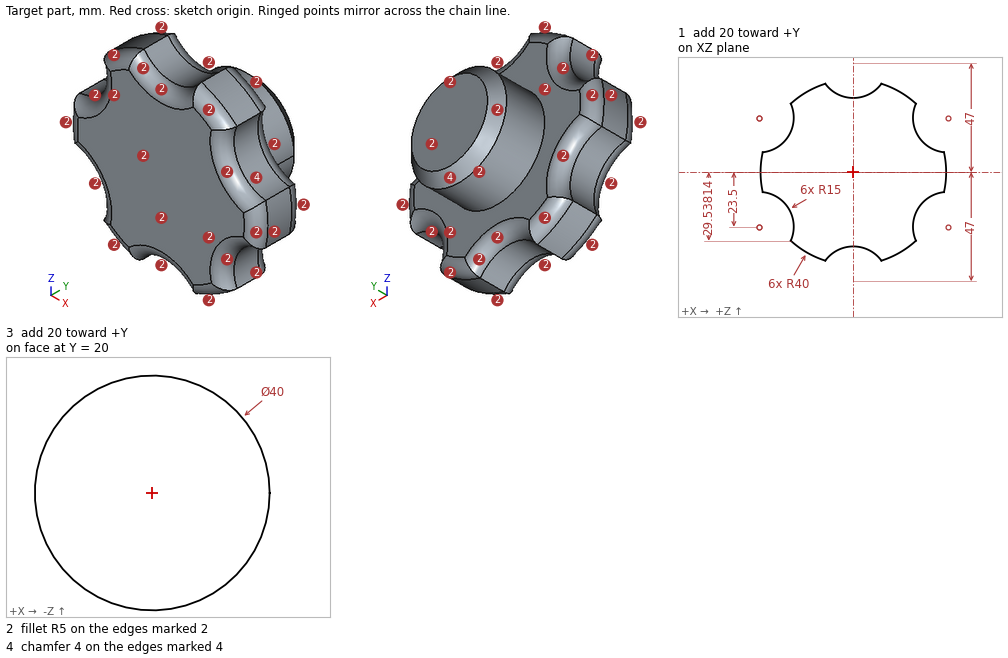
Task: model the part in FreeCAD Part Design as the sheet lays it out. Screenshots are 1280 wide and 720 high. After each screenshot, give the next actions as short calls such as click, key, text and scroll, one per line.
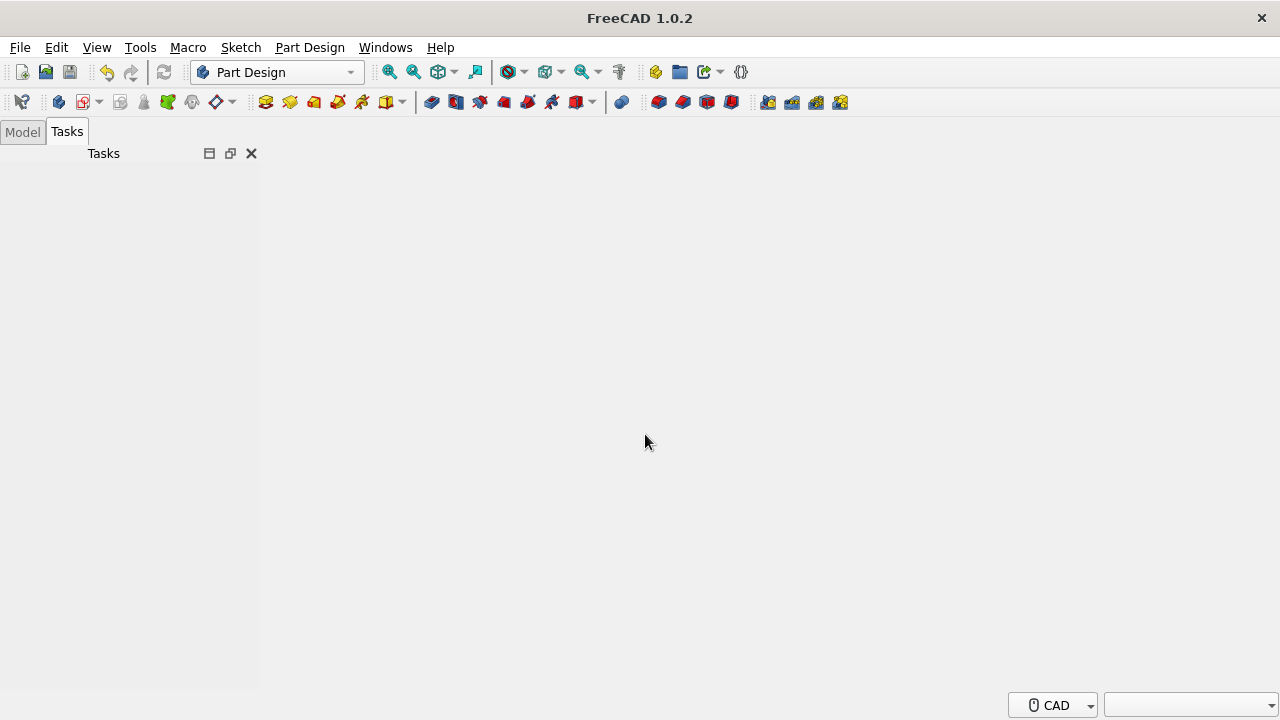
click(22, 72)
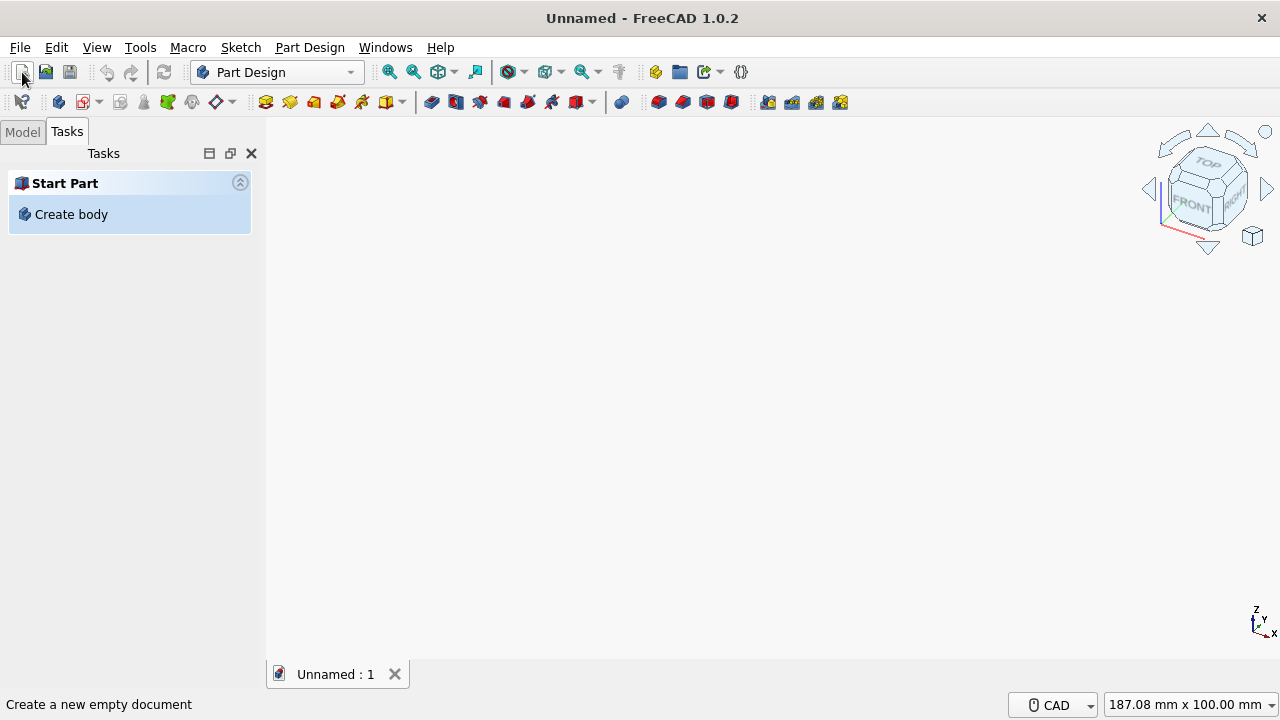
click(84, 102)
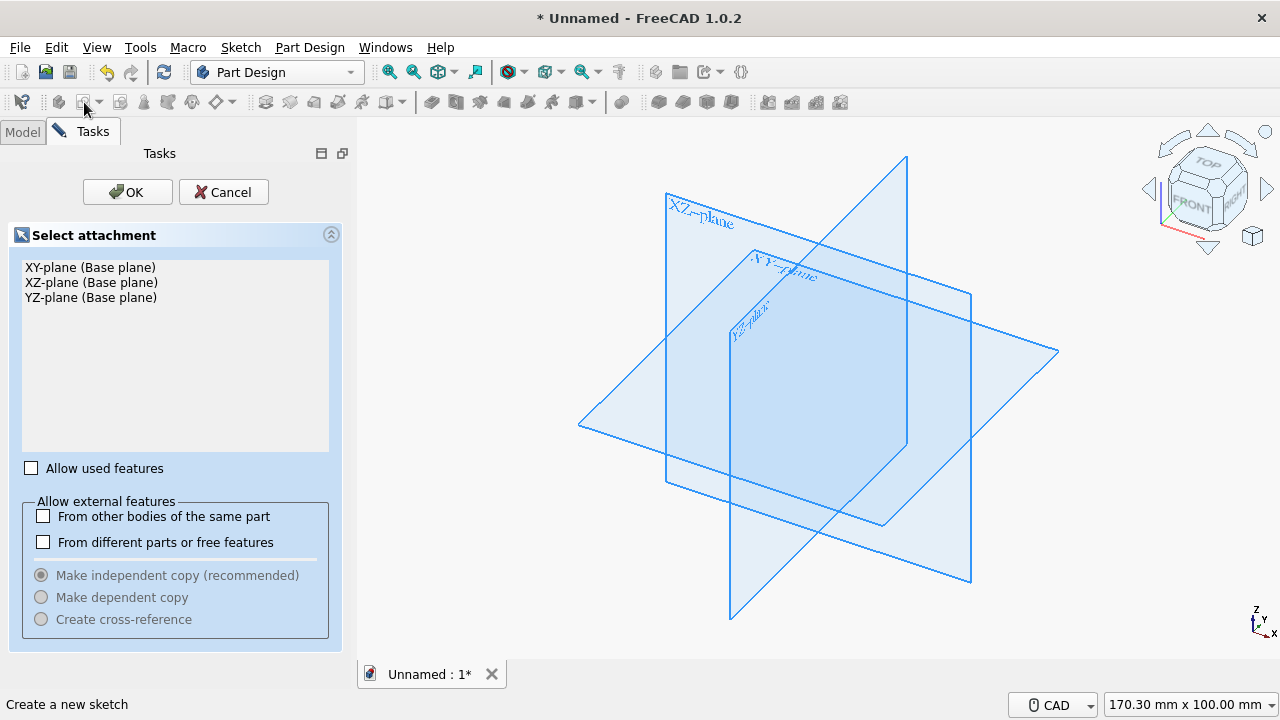
click(82, 282)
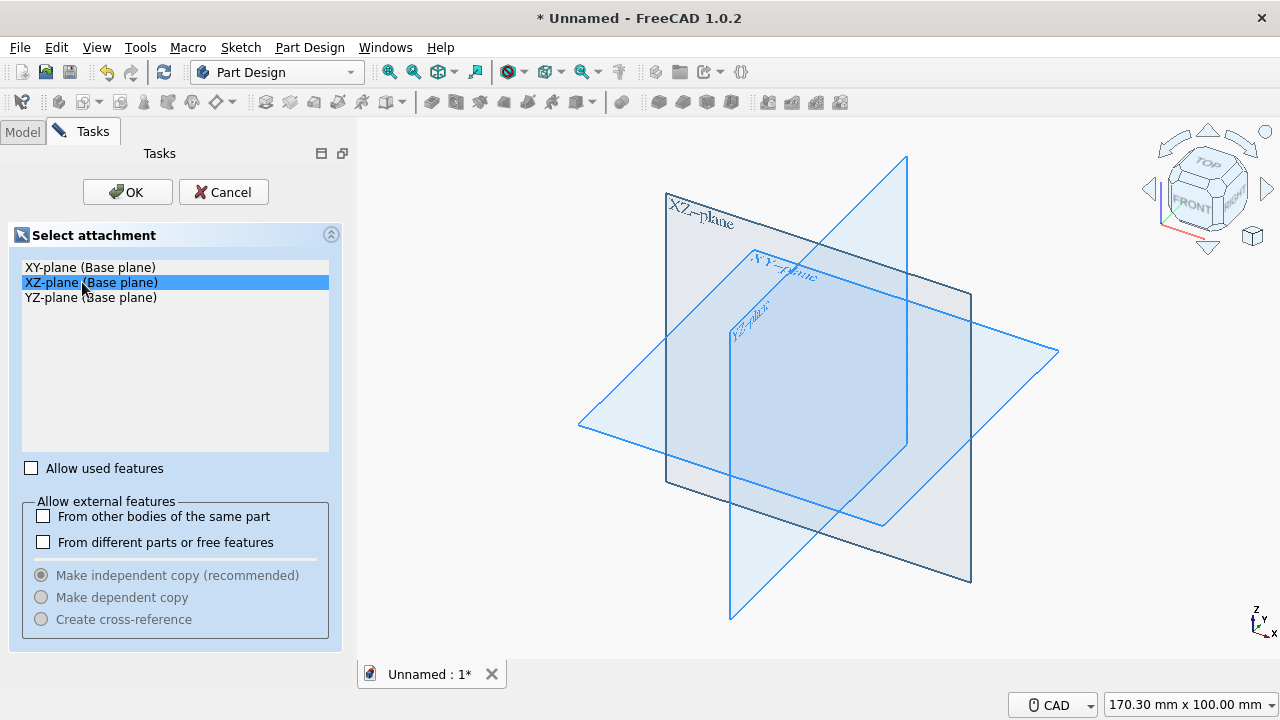
click(128, 192)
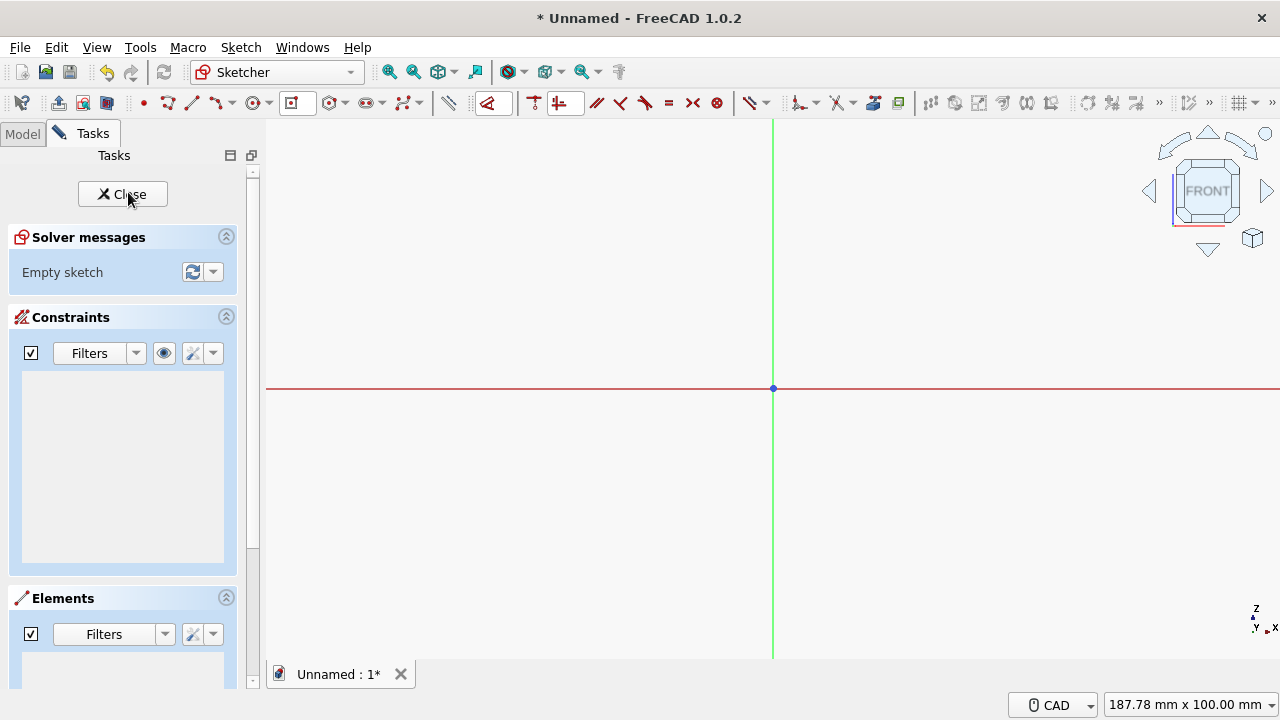
click(216, 104)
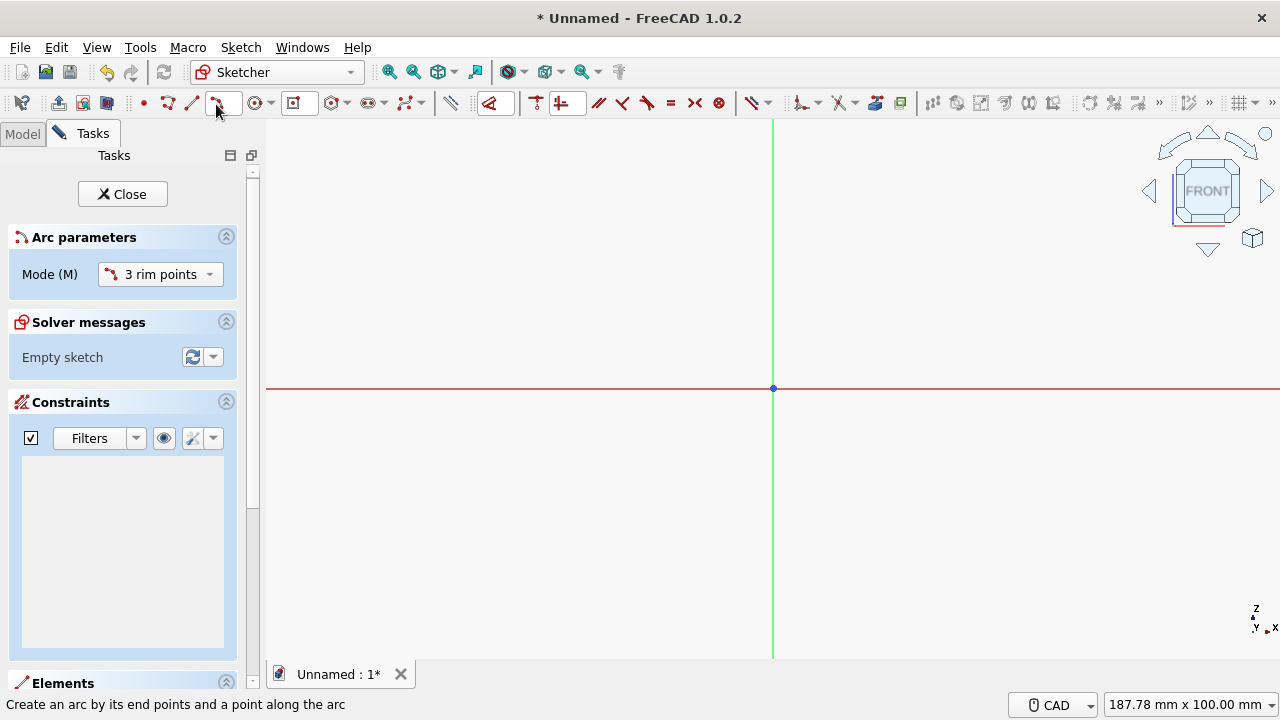
click(708, 595)
click(627, 549)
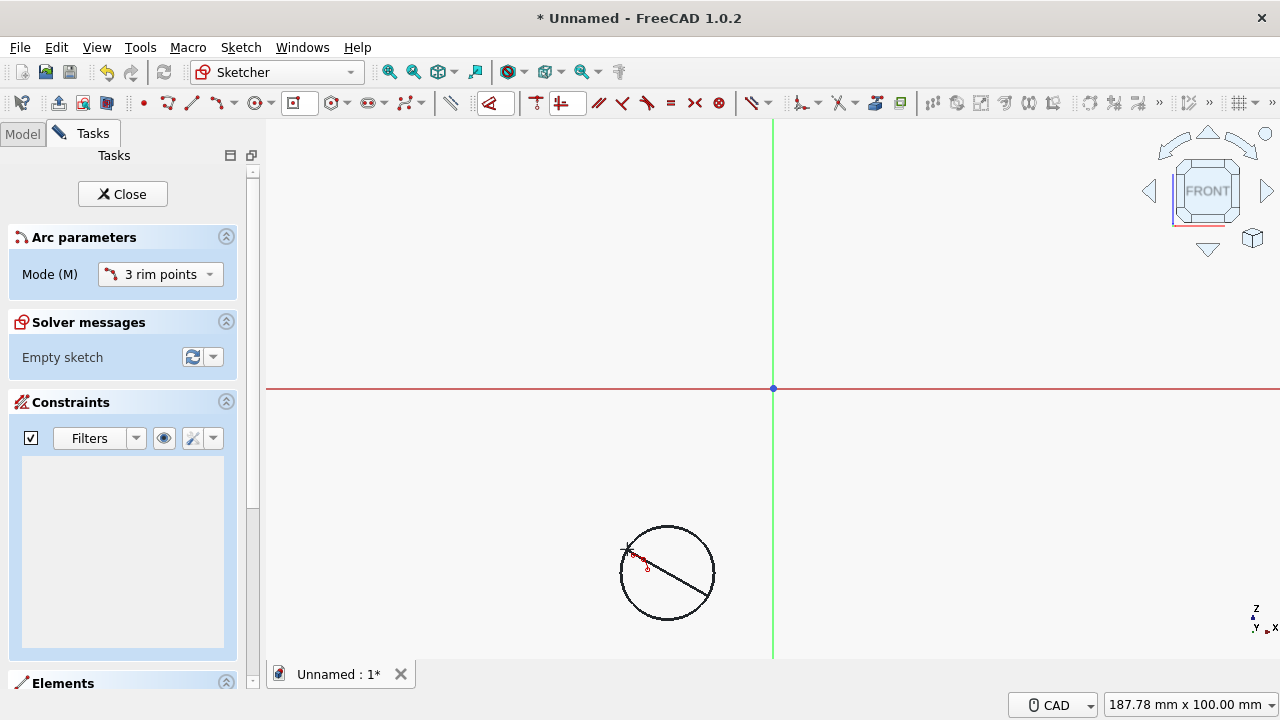
scroll(665, 576, up, 6)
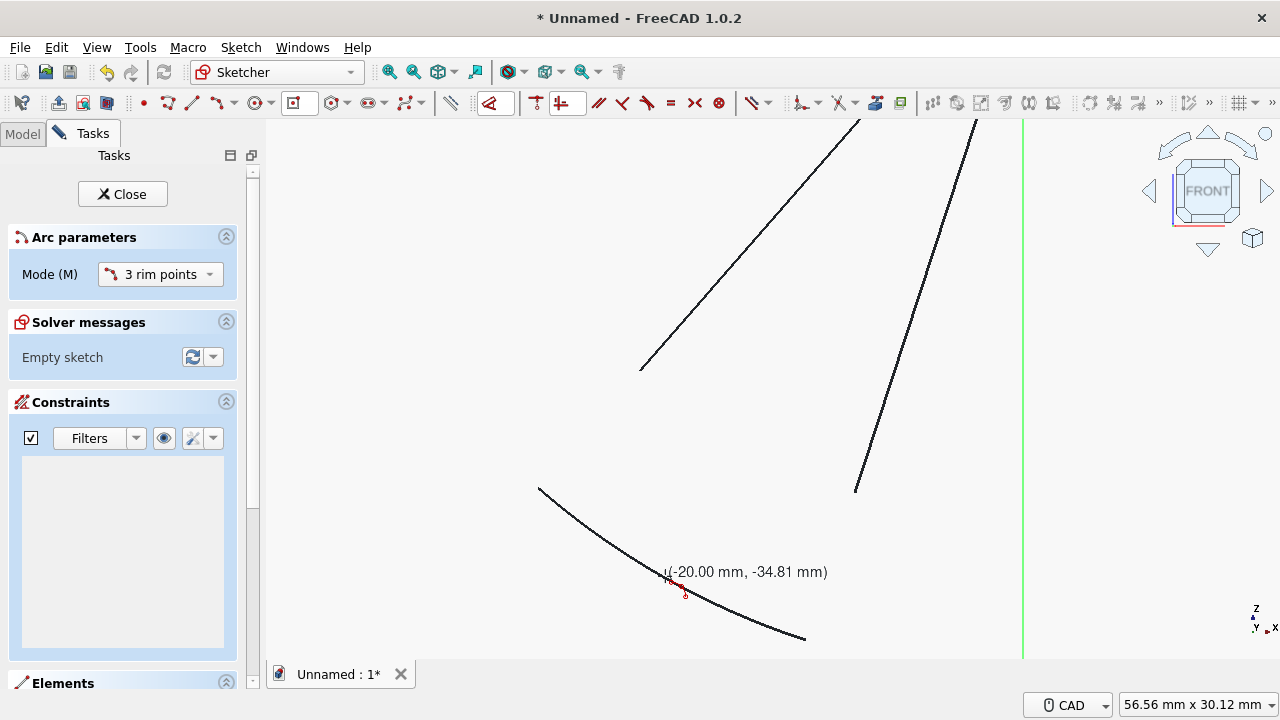
click(664, 574)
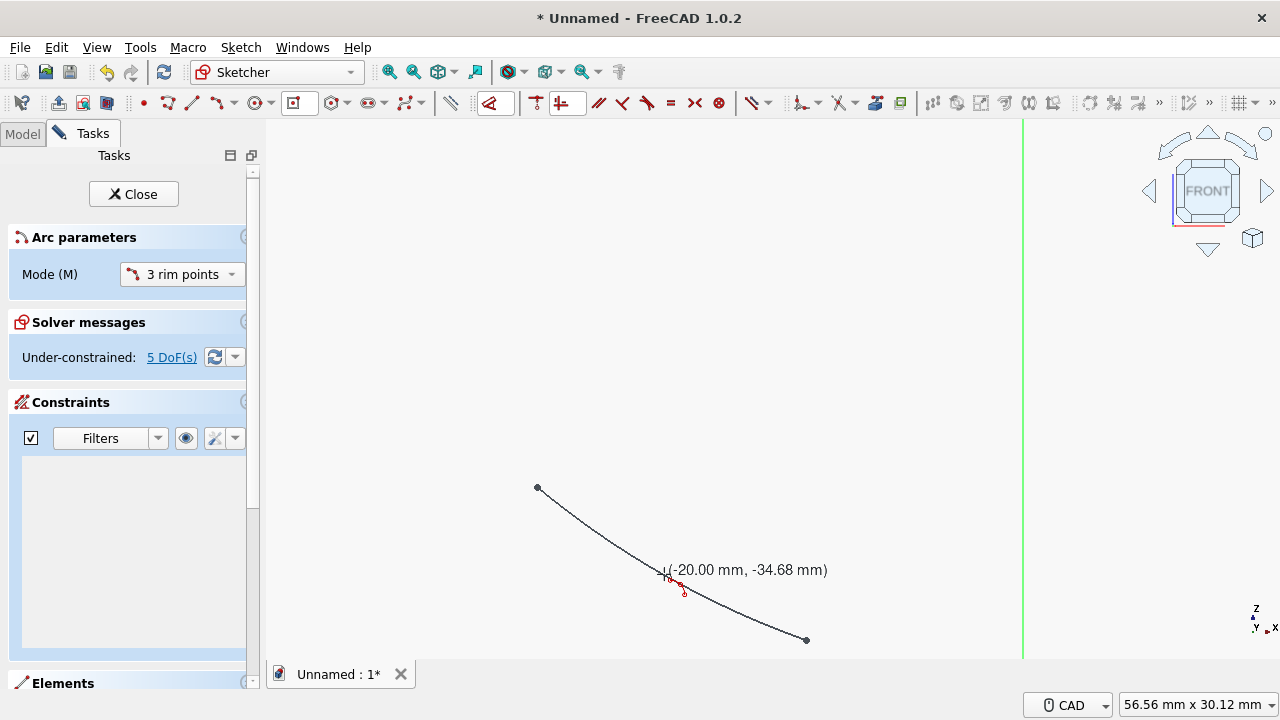
click(538, 488)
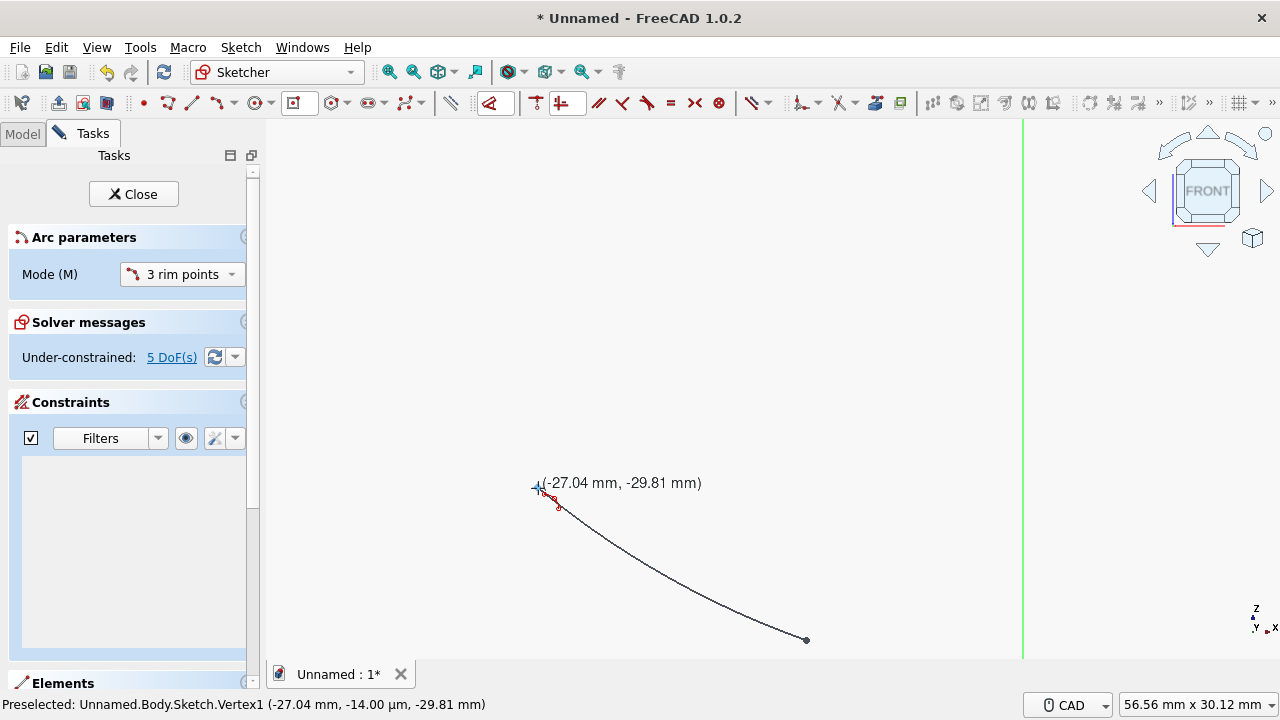
scroll(600, 532, down, 7)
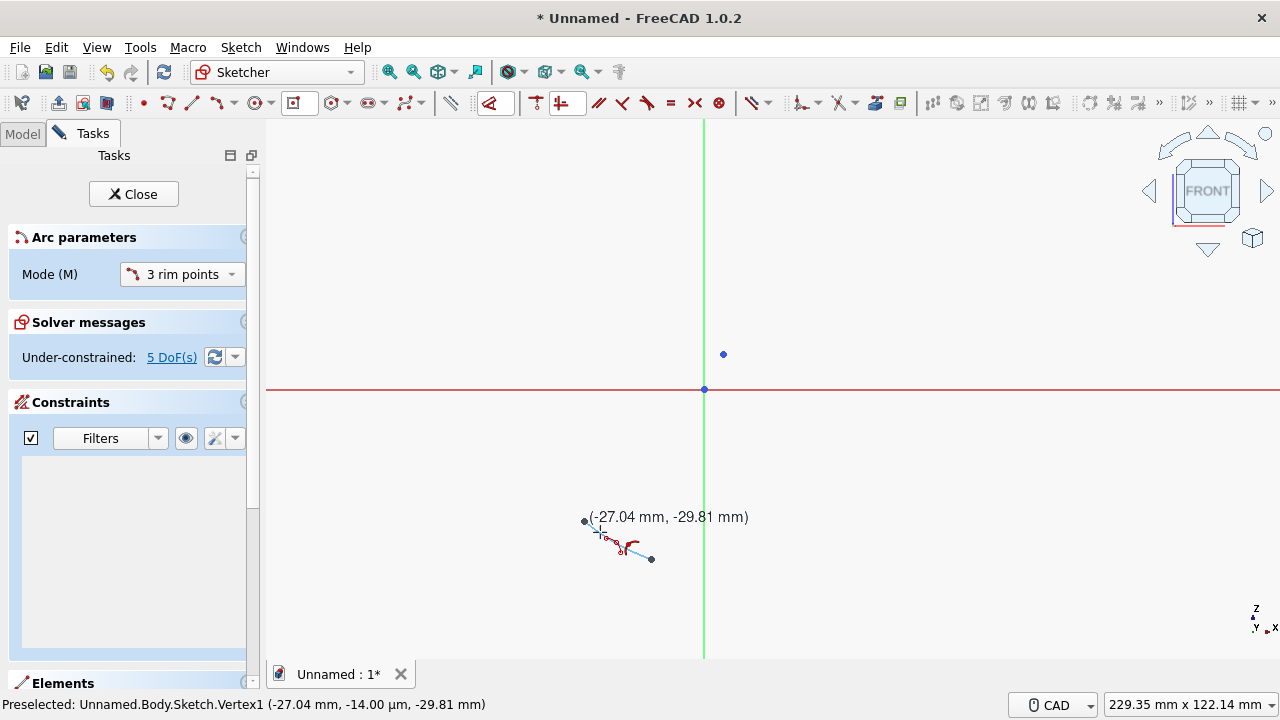
click(532, 428)
click(582, 461)